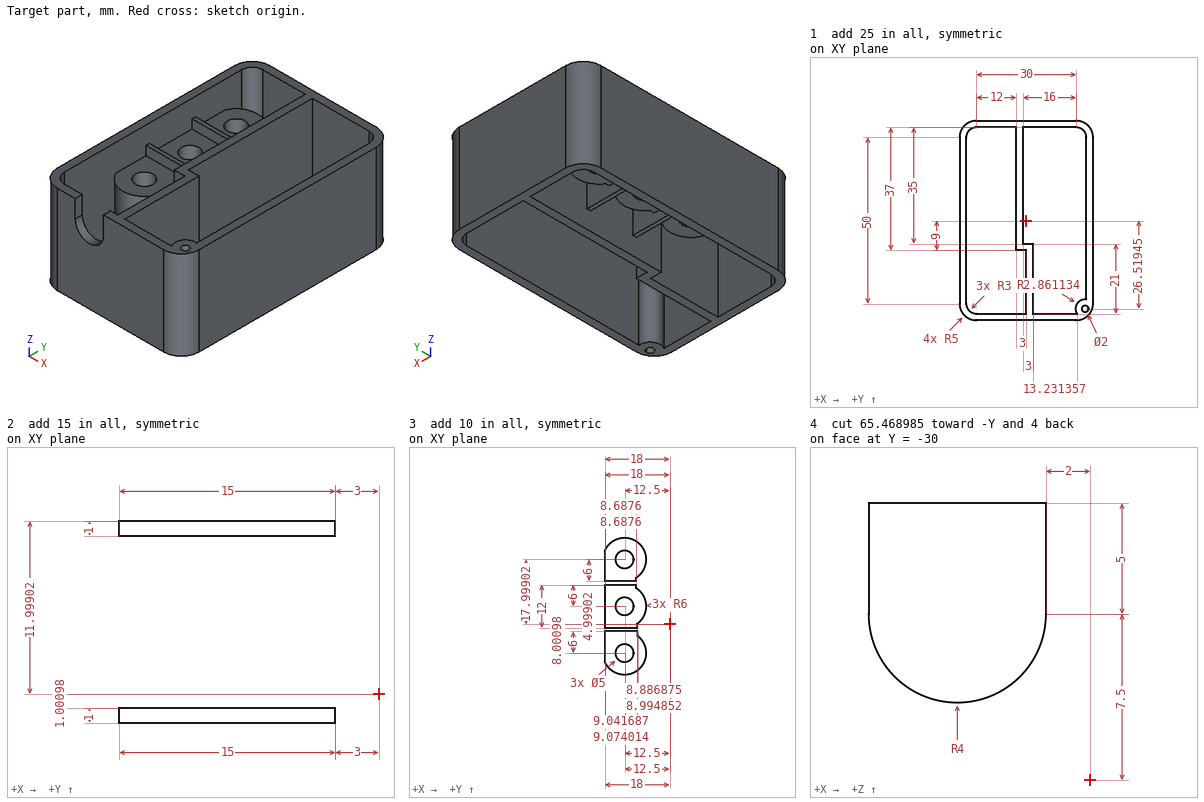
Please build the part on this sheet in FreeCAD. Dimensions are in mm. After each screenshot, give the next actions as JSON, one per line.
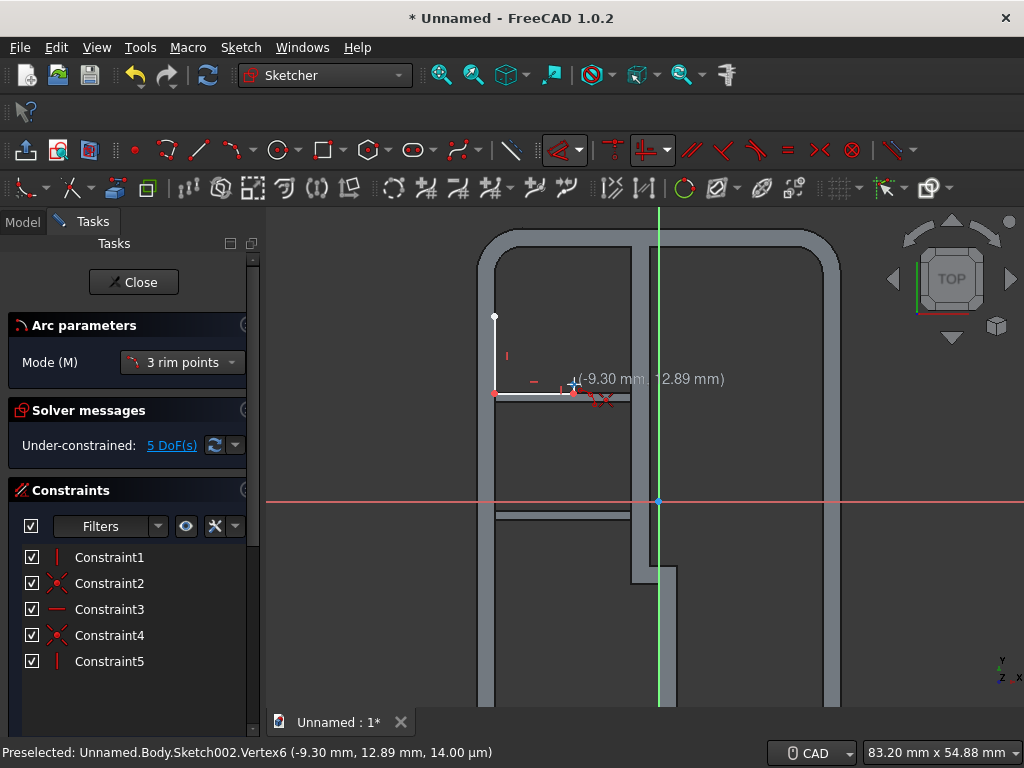
{"action": "left_click", "coordinate": [495, 317]}
{"action": "left_click", "coordinate": [581, 296]}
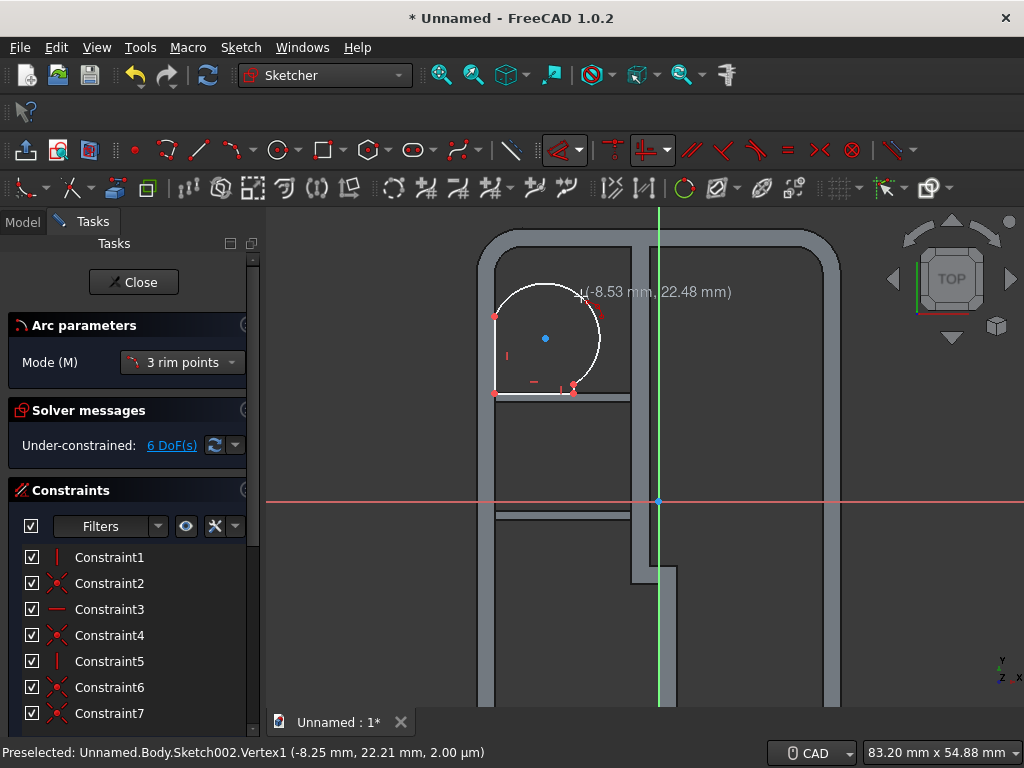
{"action": "left_click", "coordinate": [168, 150]}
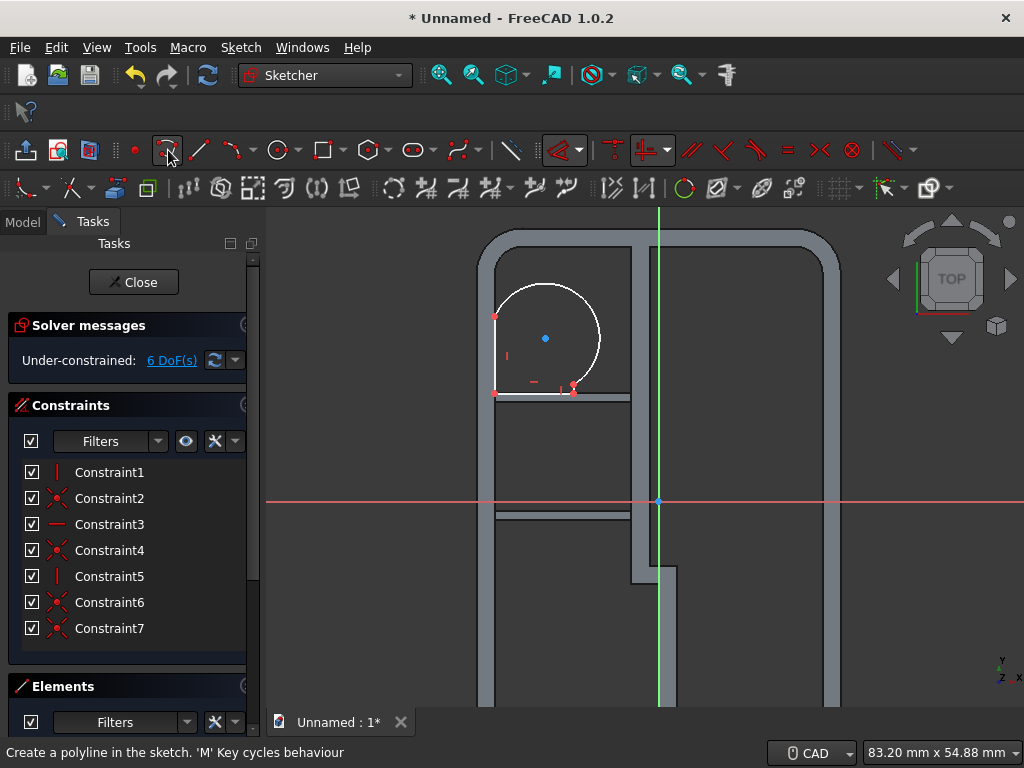
{"action": "left_click", "coordinate": [574, 410]}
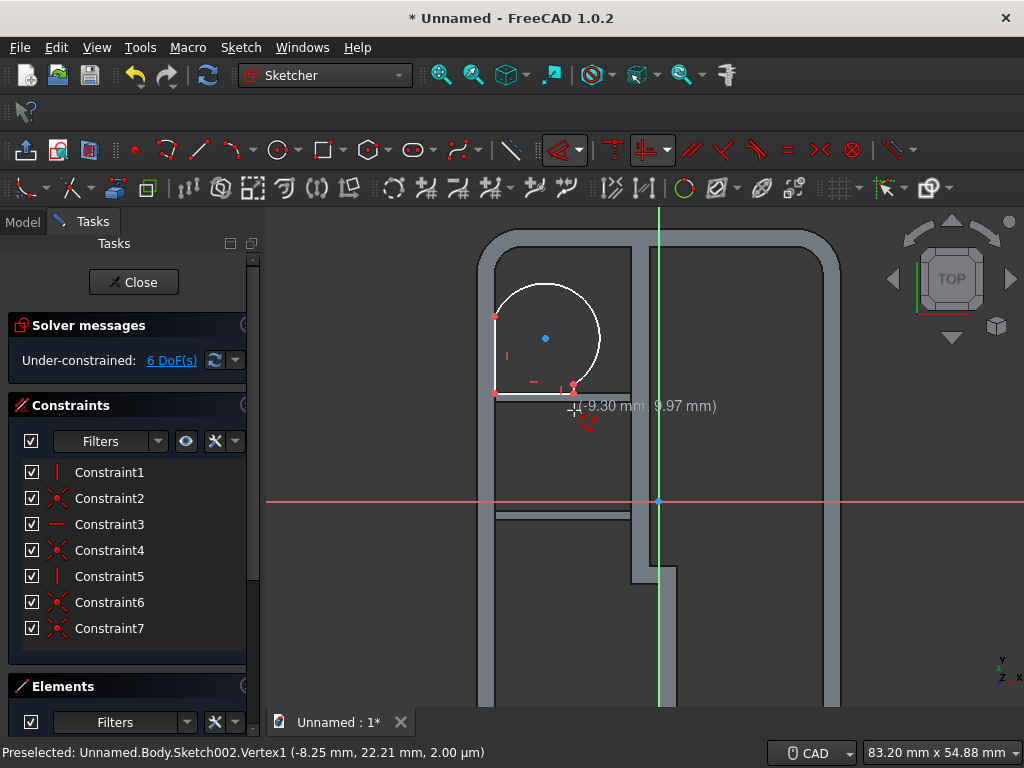
{"action": "scroll", "coordinate": [574, 402], "scroll_direction": "up", "scroll_amount": 4}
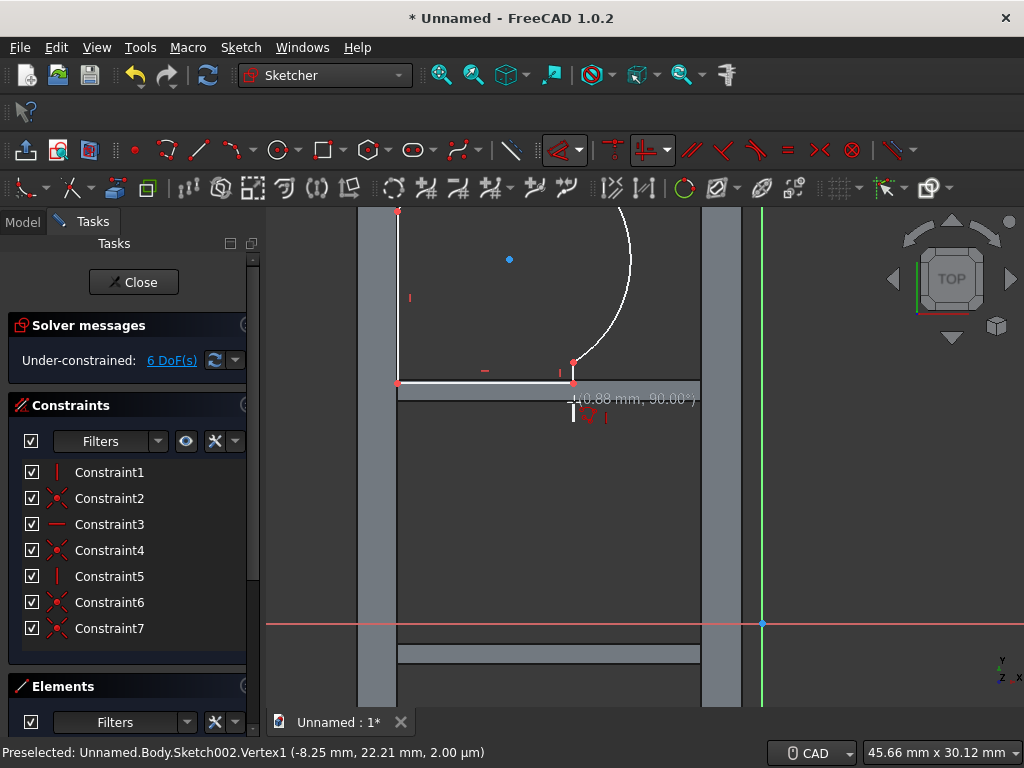
{"action": "left_click", "coordinate": [574, 401]}
{"action": "left_click", "coordinate": [397, 401]}
{"action": "left_click", "coordinate": [397, 644]}
{"action": "left_click", "coordinate": [580, 644]}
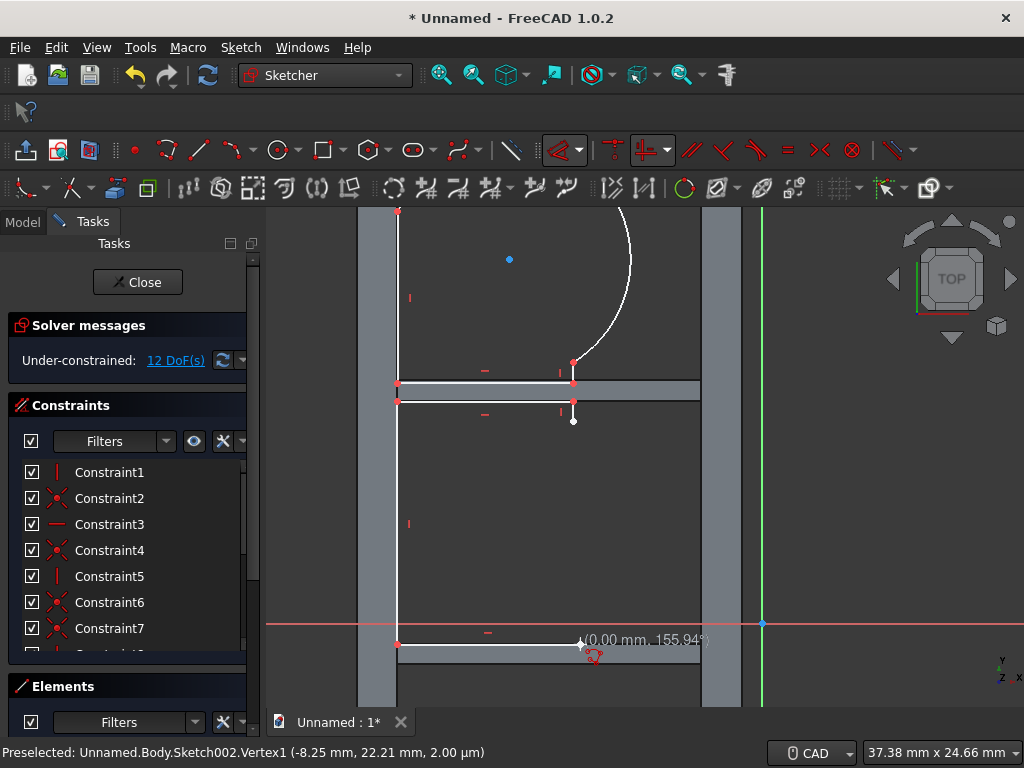
{"action": "scroll", "coordinate": [580, 621], "scroll_direction": "up", "scroll_amount": 10}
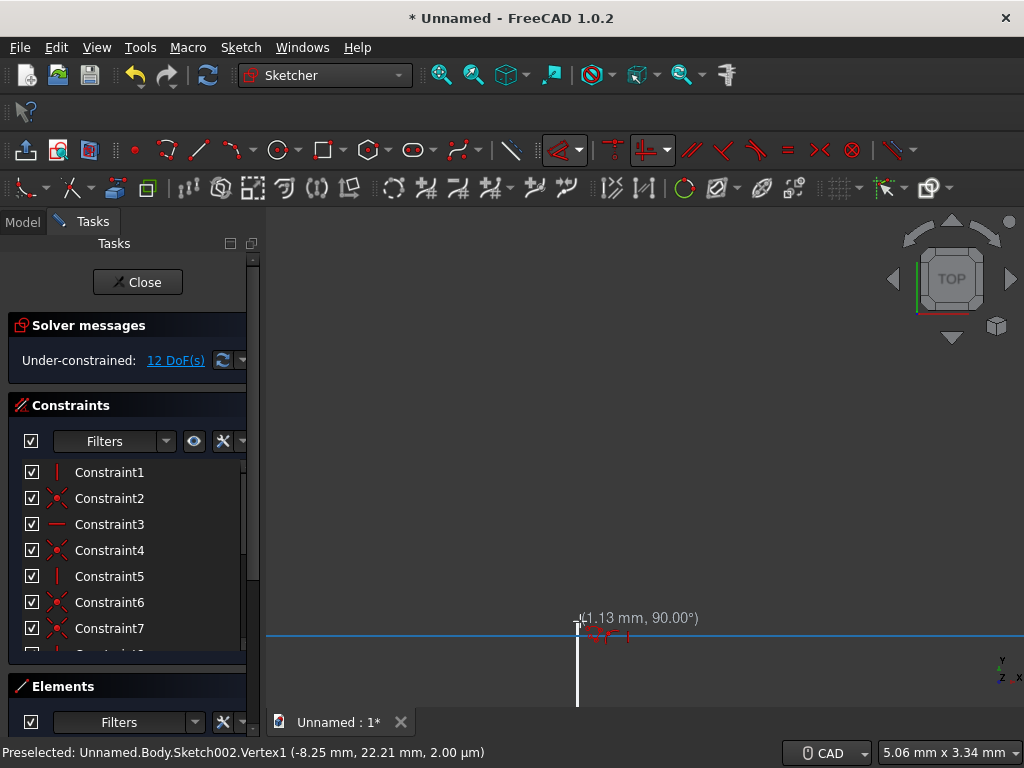
{"action": "left_click", "coordinate": [568, 616]}
{"action": "right_click", "coordinate": [568, 616]}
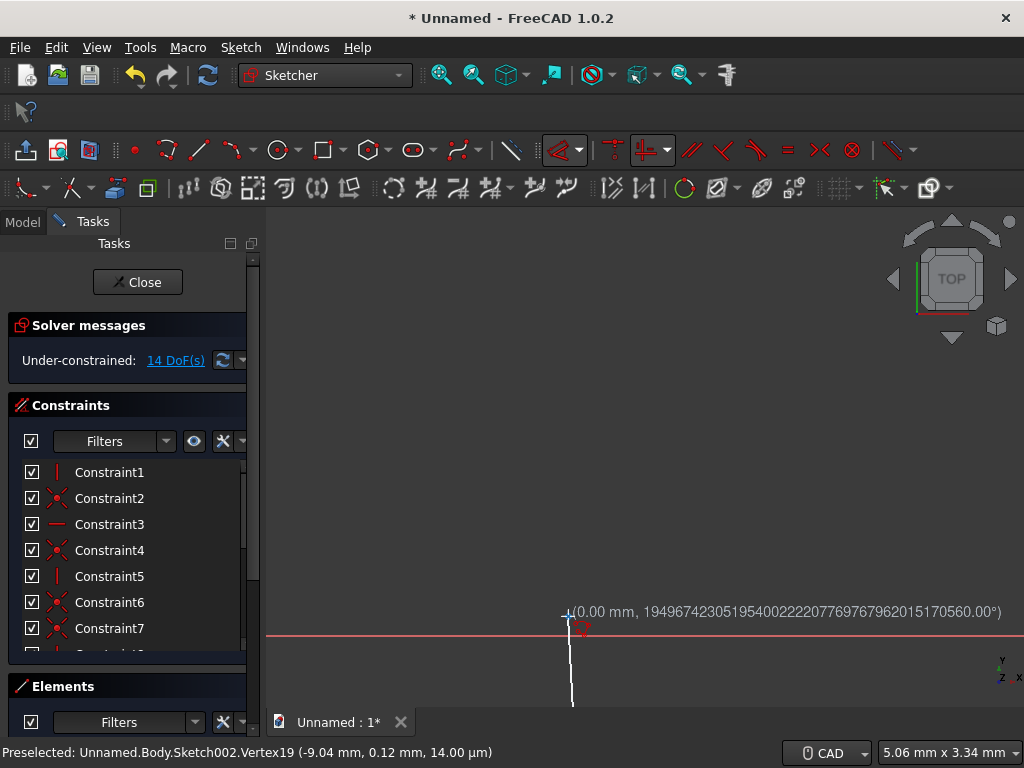
{"action": "left_click", "coordinate": [232, 150]}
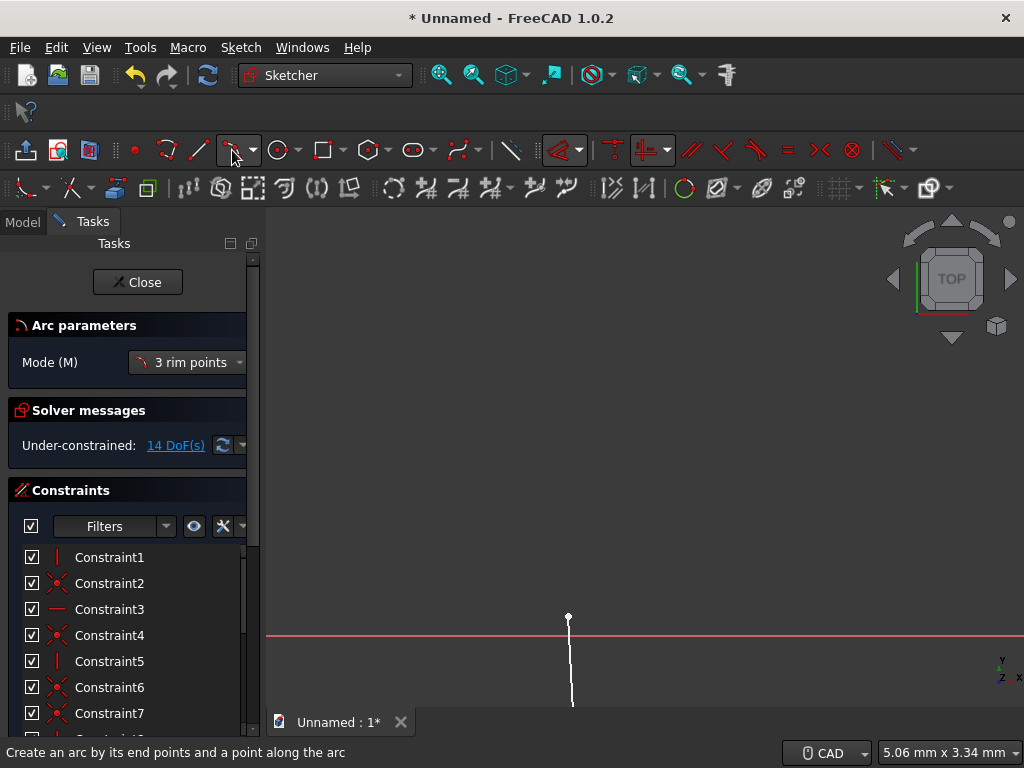
{"action": "left_click", "coordinate": [568, 617]}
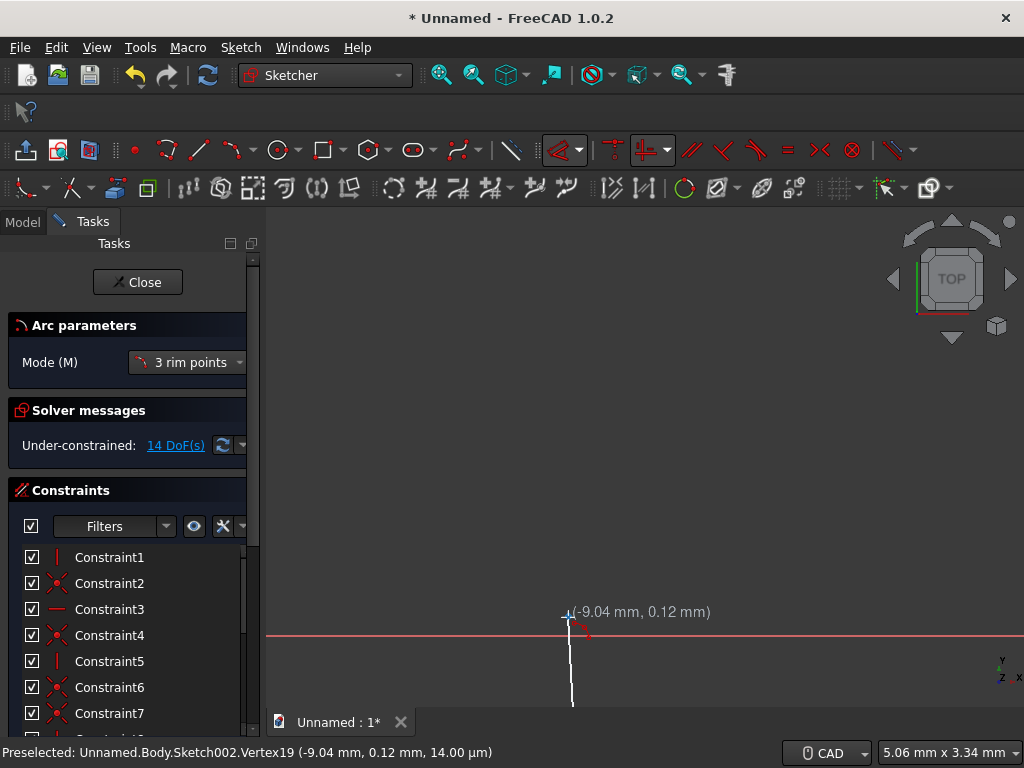
{"action": "scroll", "coordinate": [577, 493], "scroll_direction": "down", "scroll_amount": 14}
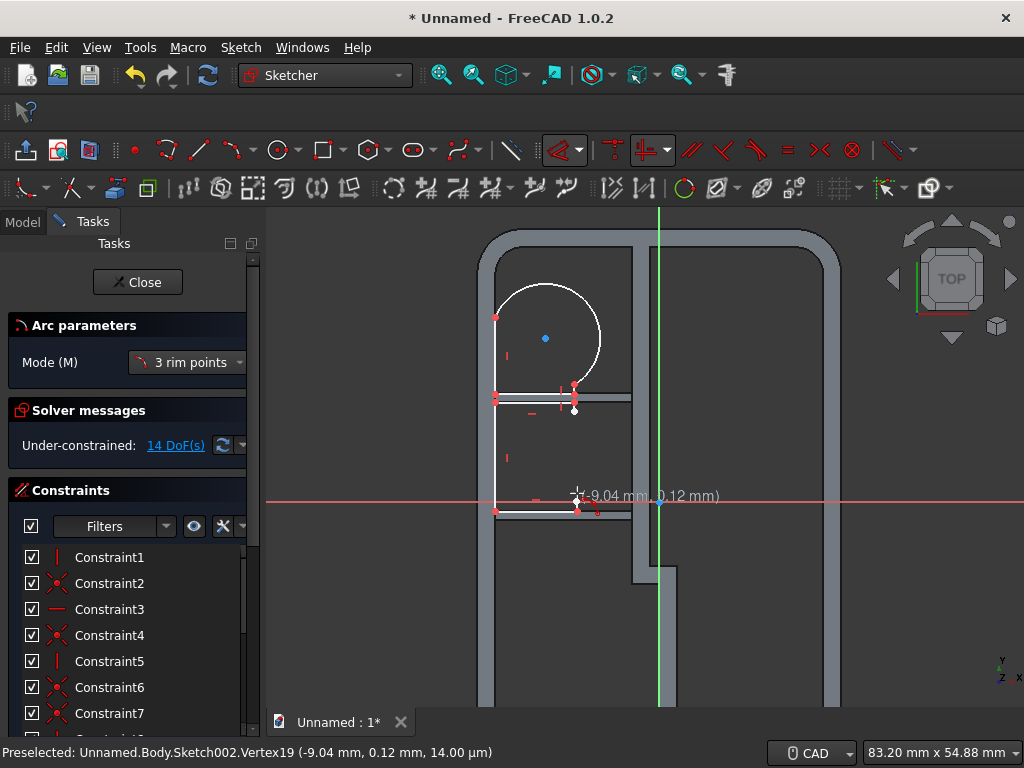
{"action": "scroll", "coordinate": [574, 410], "scroll_direction": "up", "scroll_amount": 7}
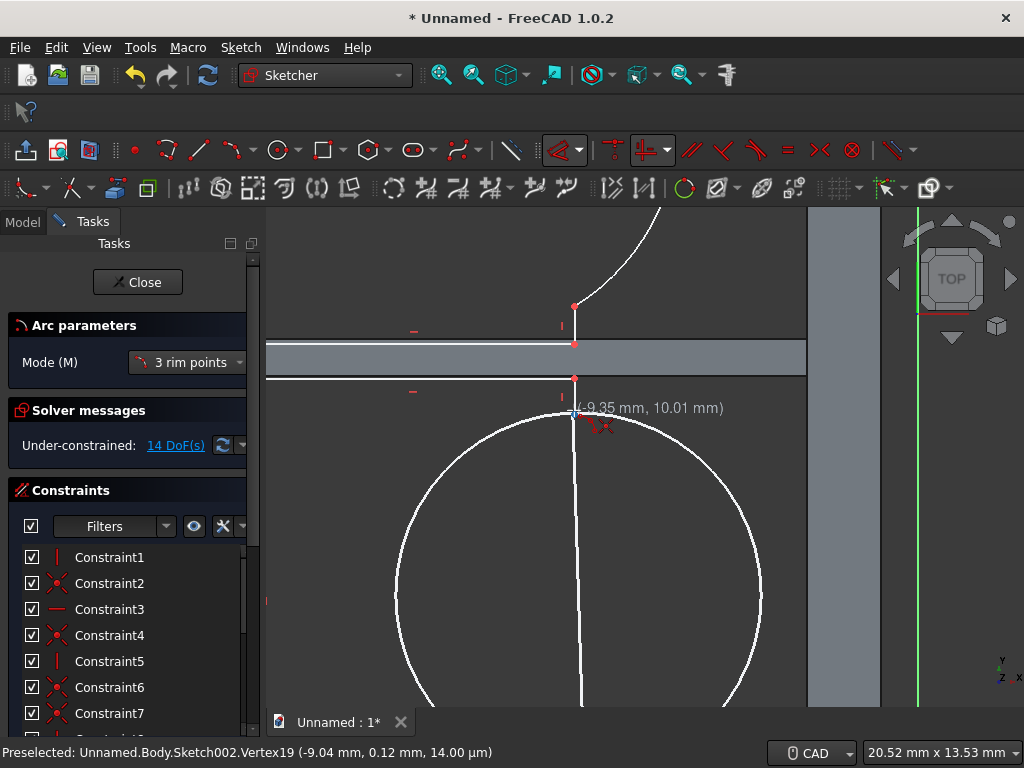
{"action": "left_click", "coordinate": [575, 414]}